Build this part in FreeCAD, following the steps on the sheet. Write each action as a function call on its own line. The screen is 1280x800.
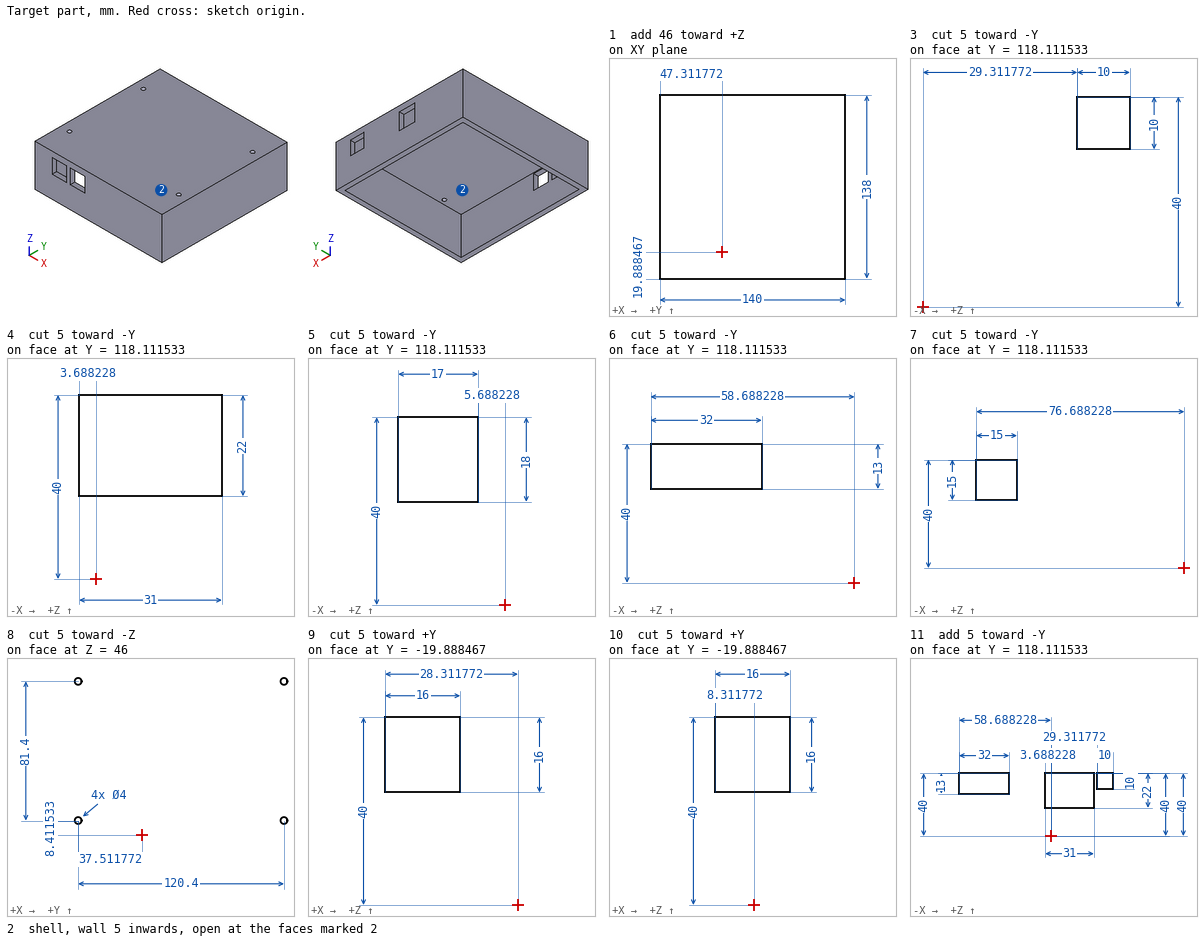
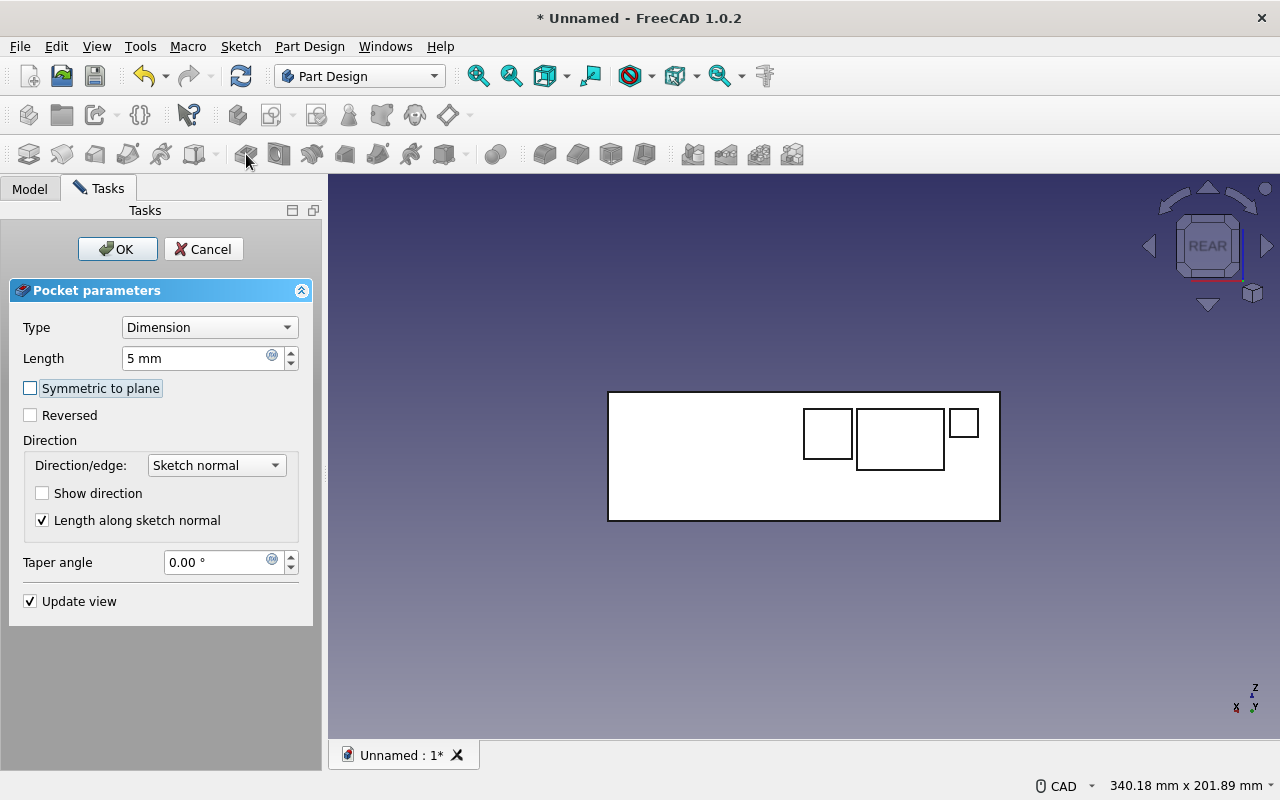
click(118, 249)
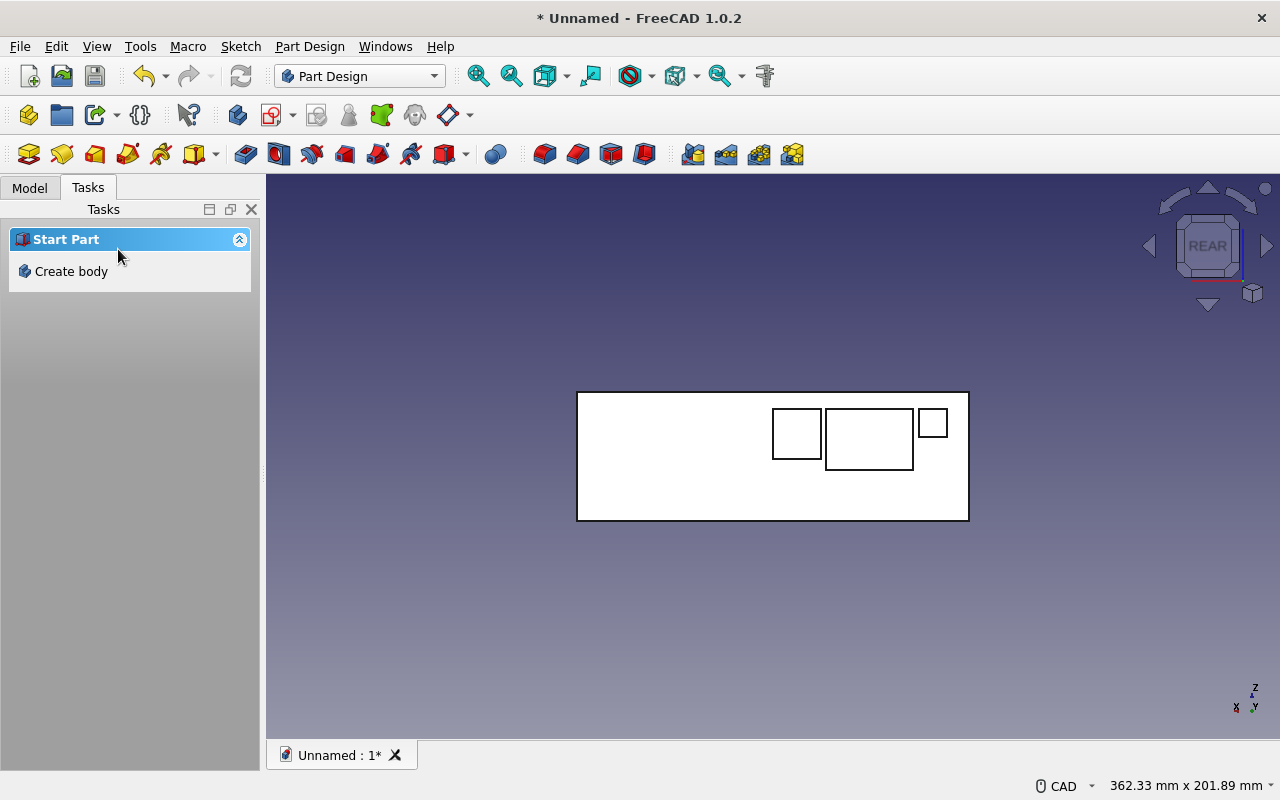
key(v)
key(f)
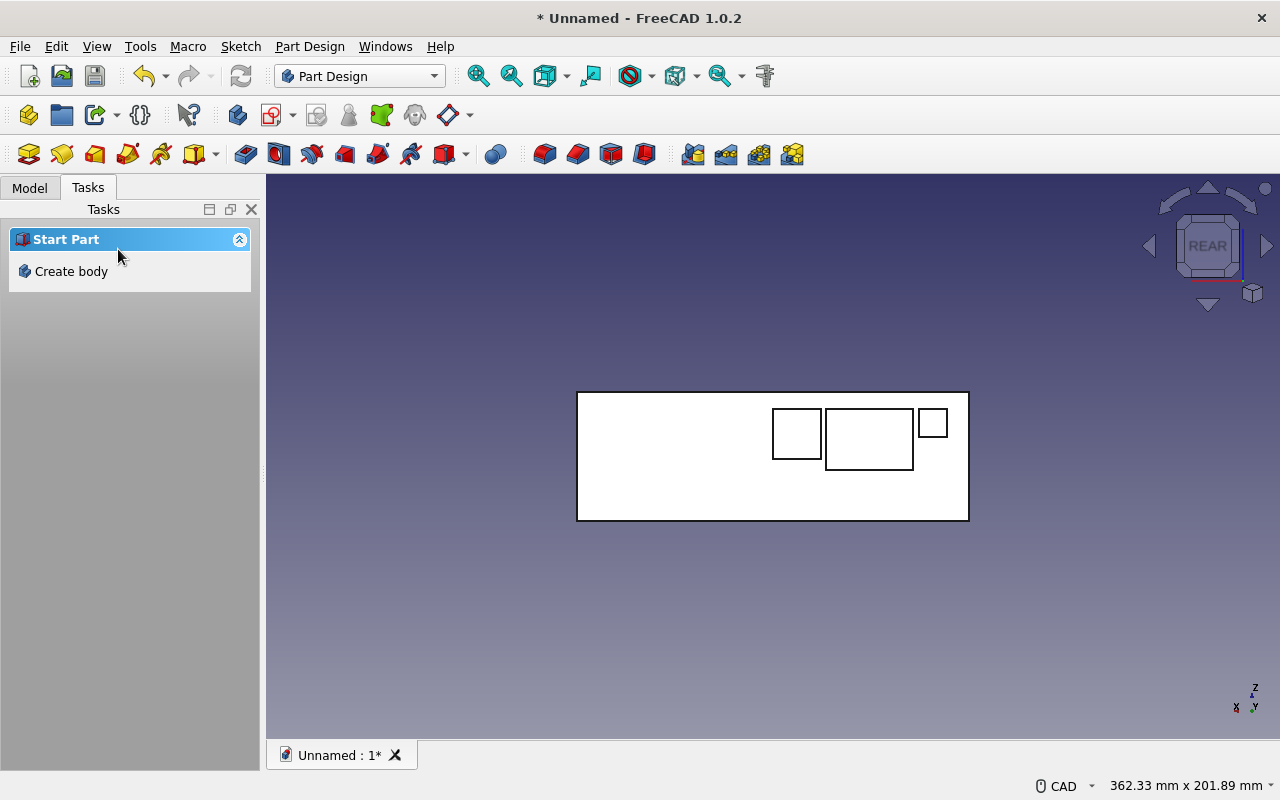
click(661, 455)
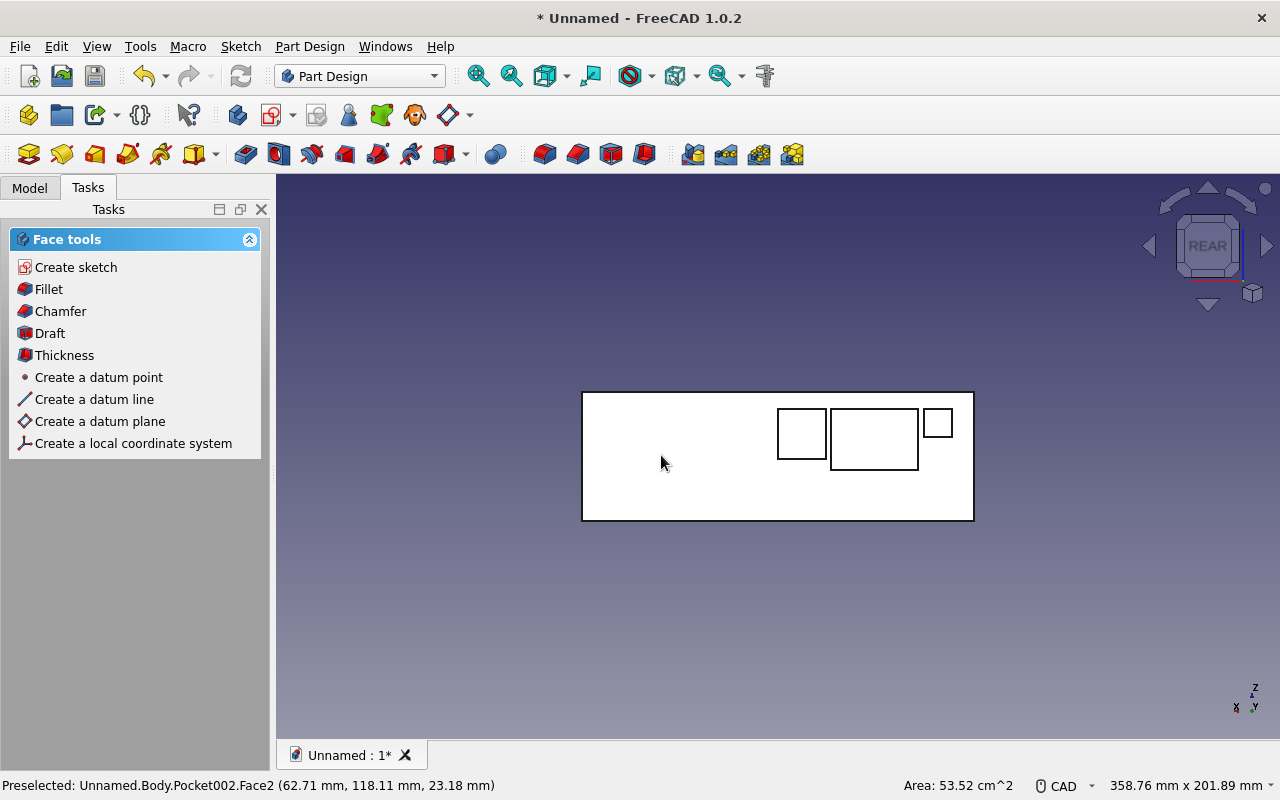
click(270, 116)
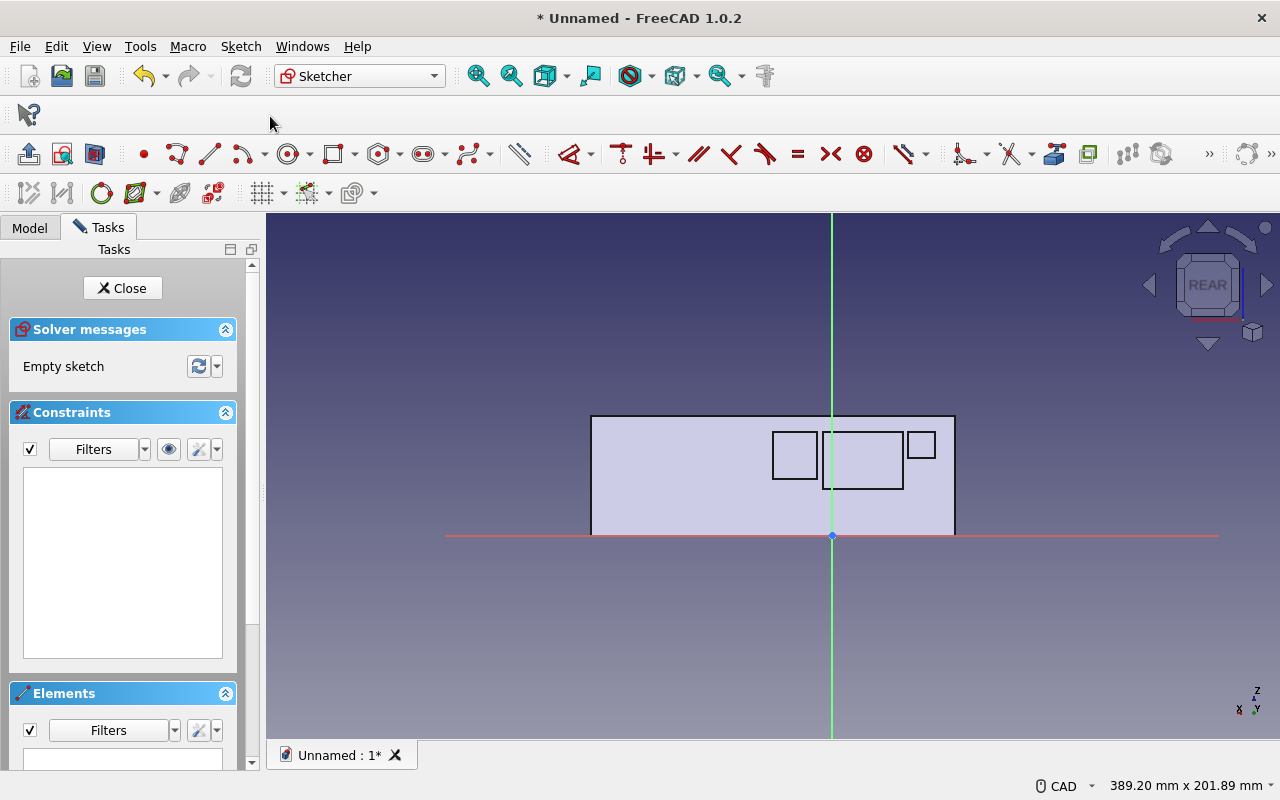
scroll(778, 487, up, 6)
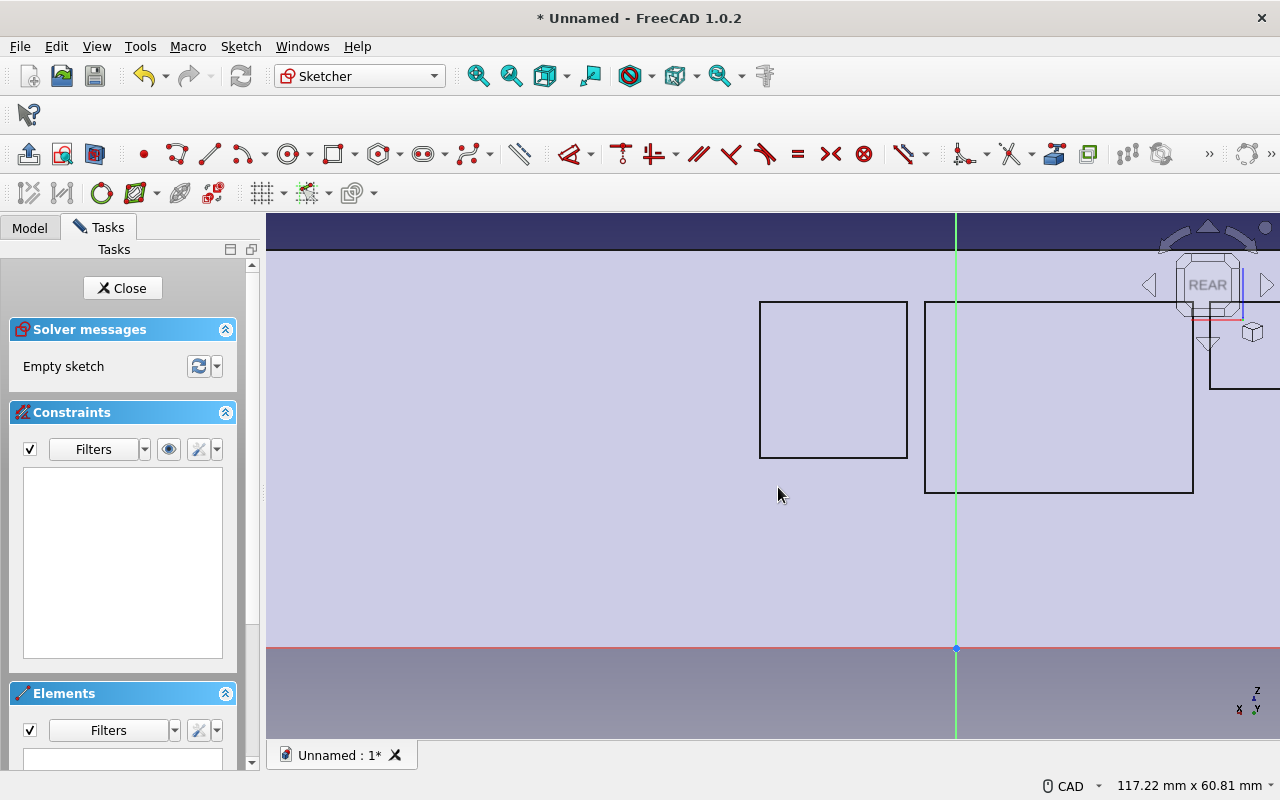
key(g)
key(r)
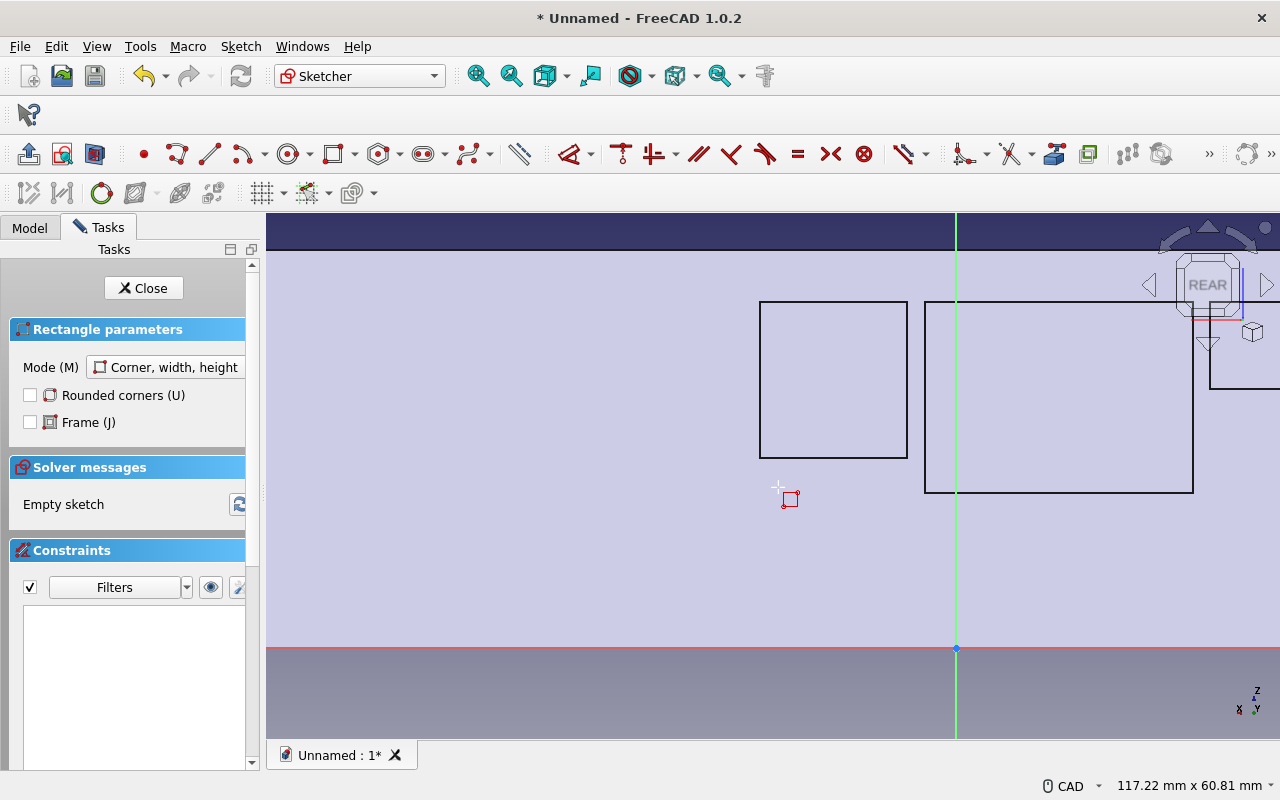
click(449, 302)
move(726, 415)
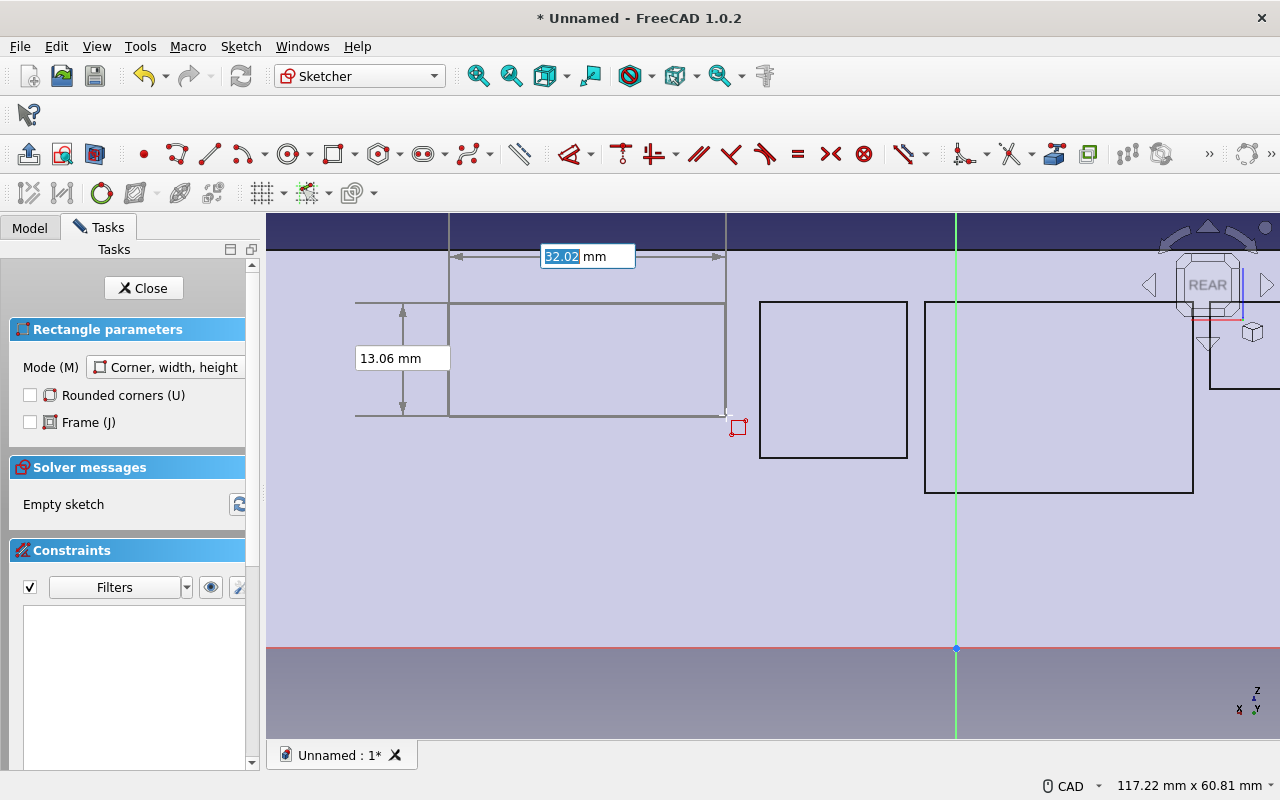
text(32)
key(Tab)
text(13)
key(Return)
key(Escape)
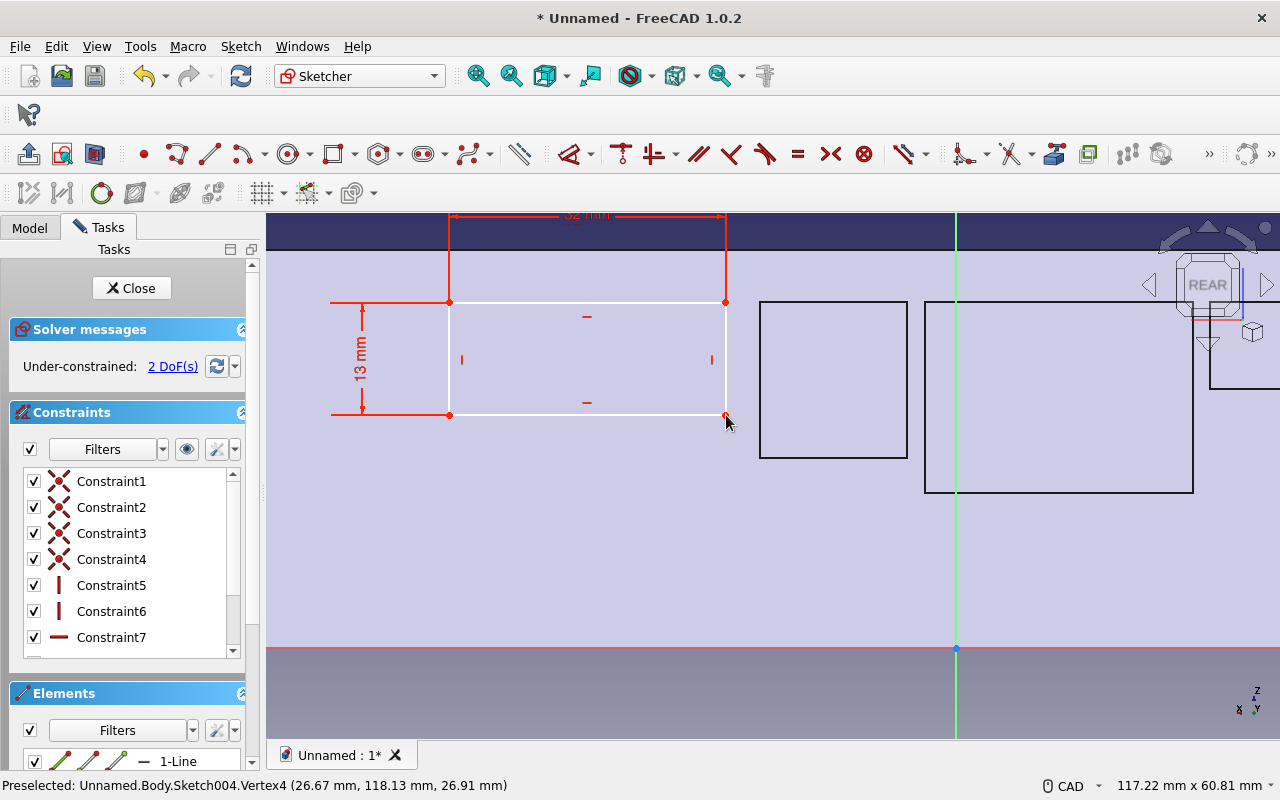
key(d)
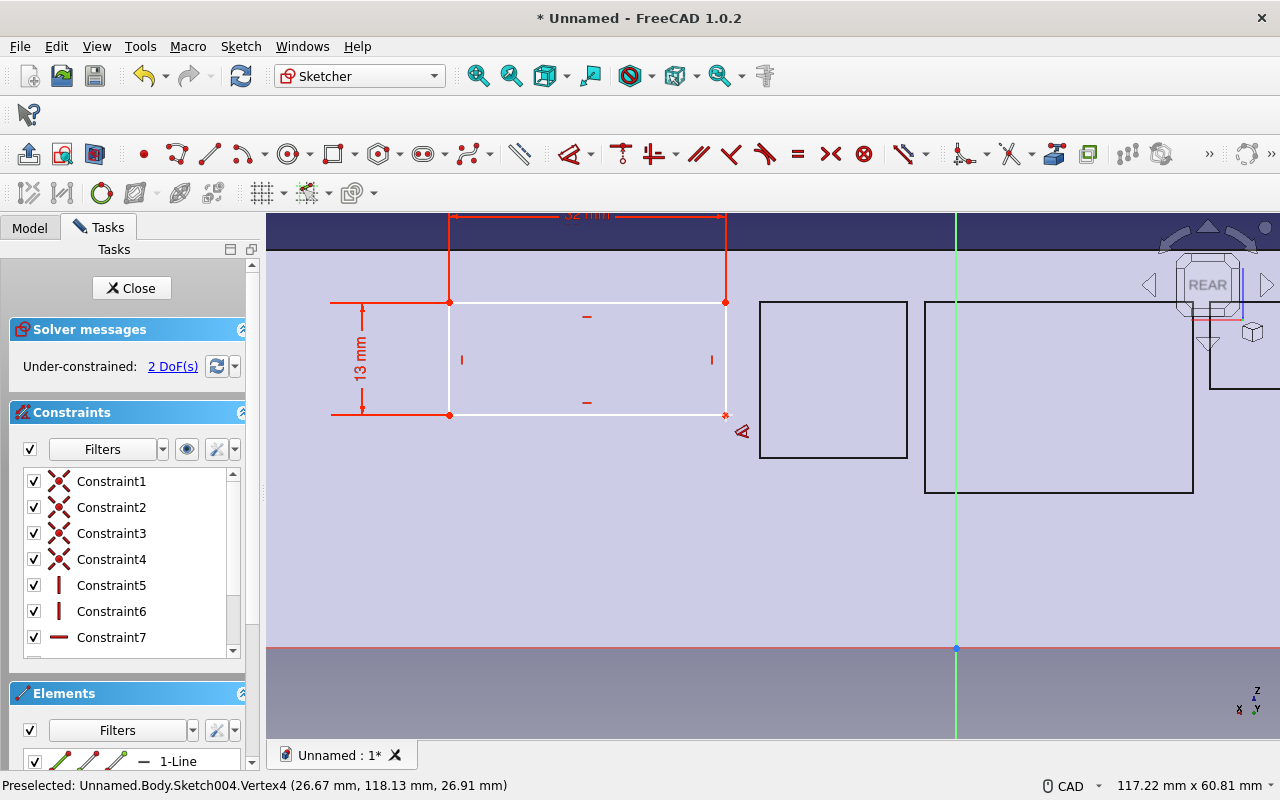
click(449, 303)
click(990, 476)